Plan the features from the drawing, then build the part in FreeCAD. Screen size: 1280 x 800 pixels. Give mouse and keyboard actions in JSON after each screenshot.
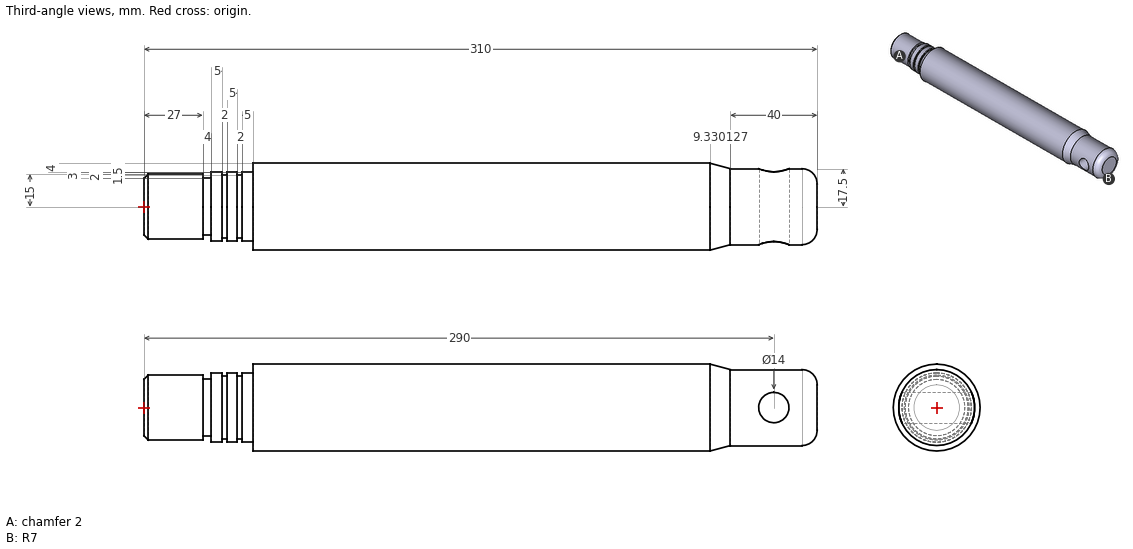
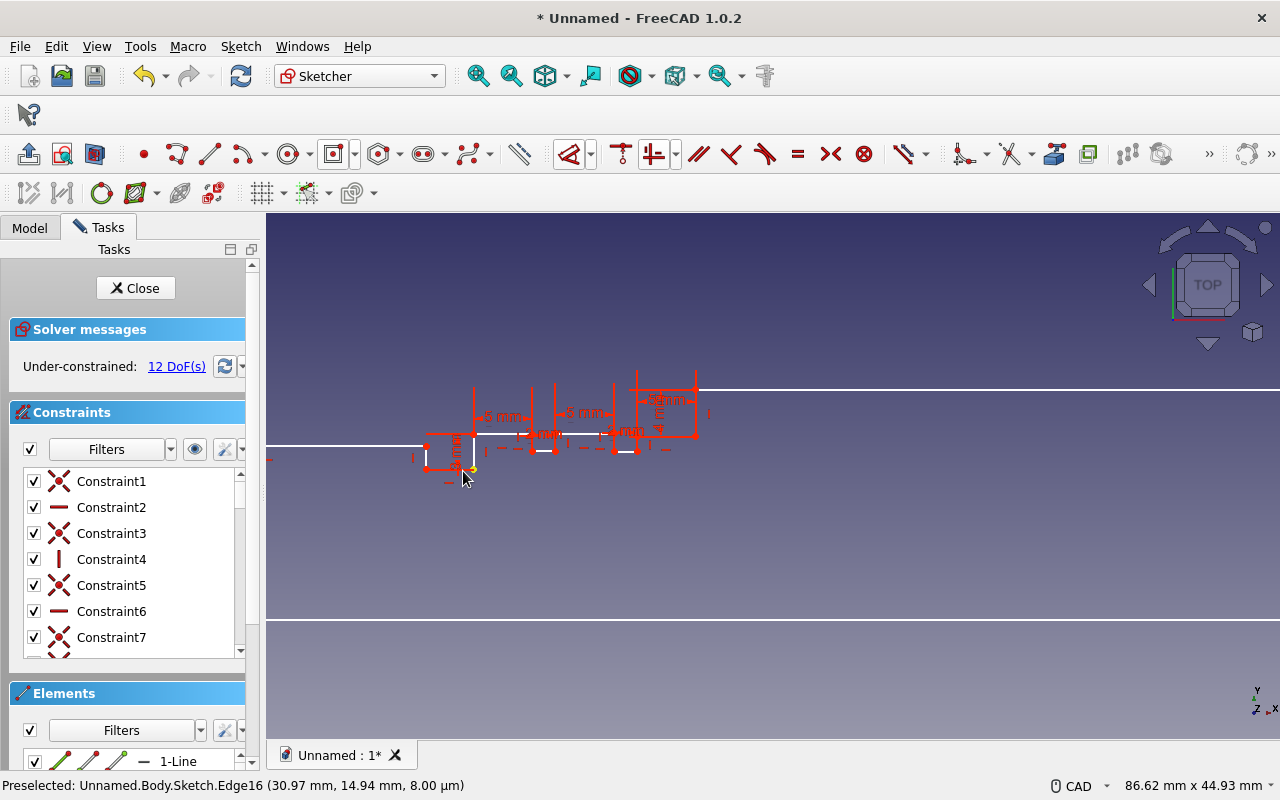
{"action": "left_click", "coordinate": [459, 470]}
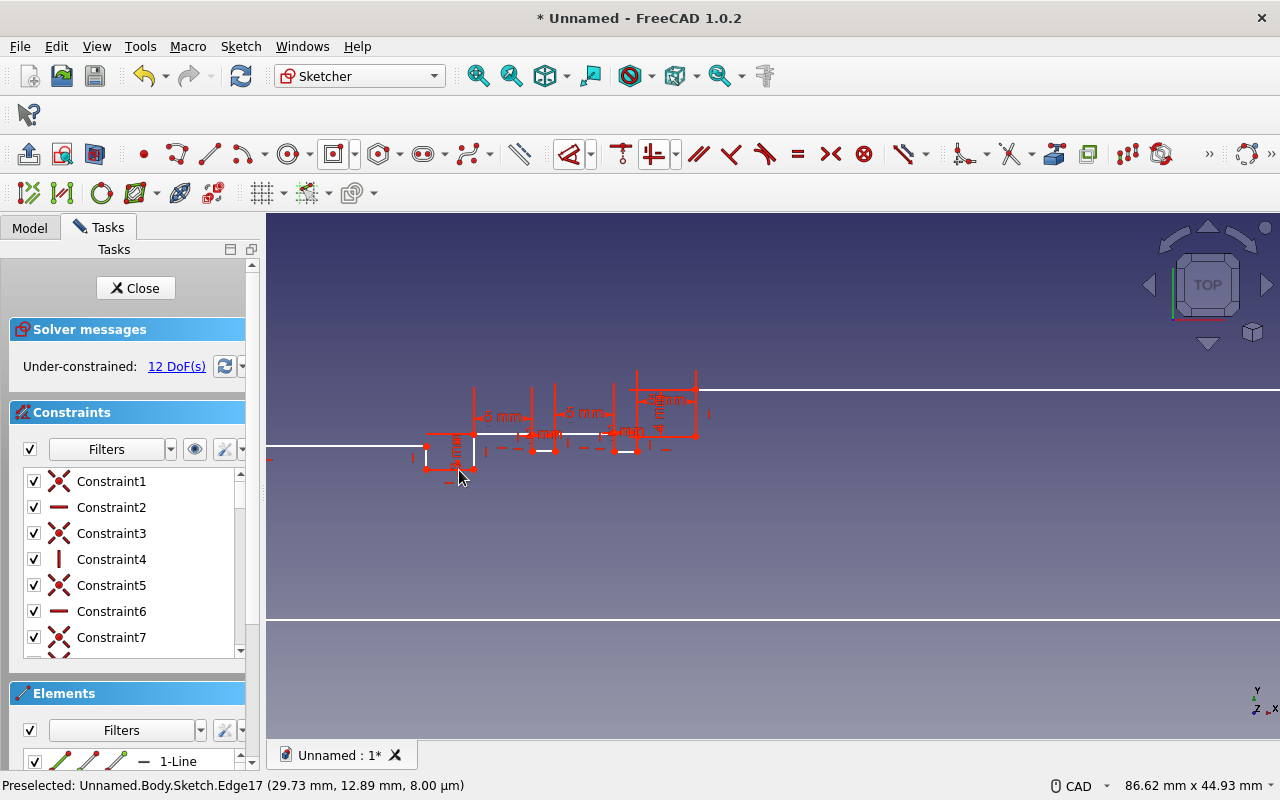
{"action": "key", "text": "l"}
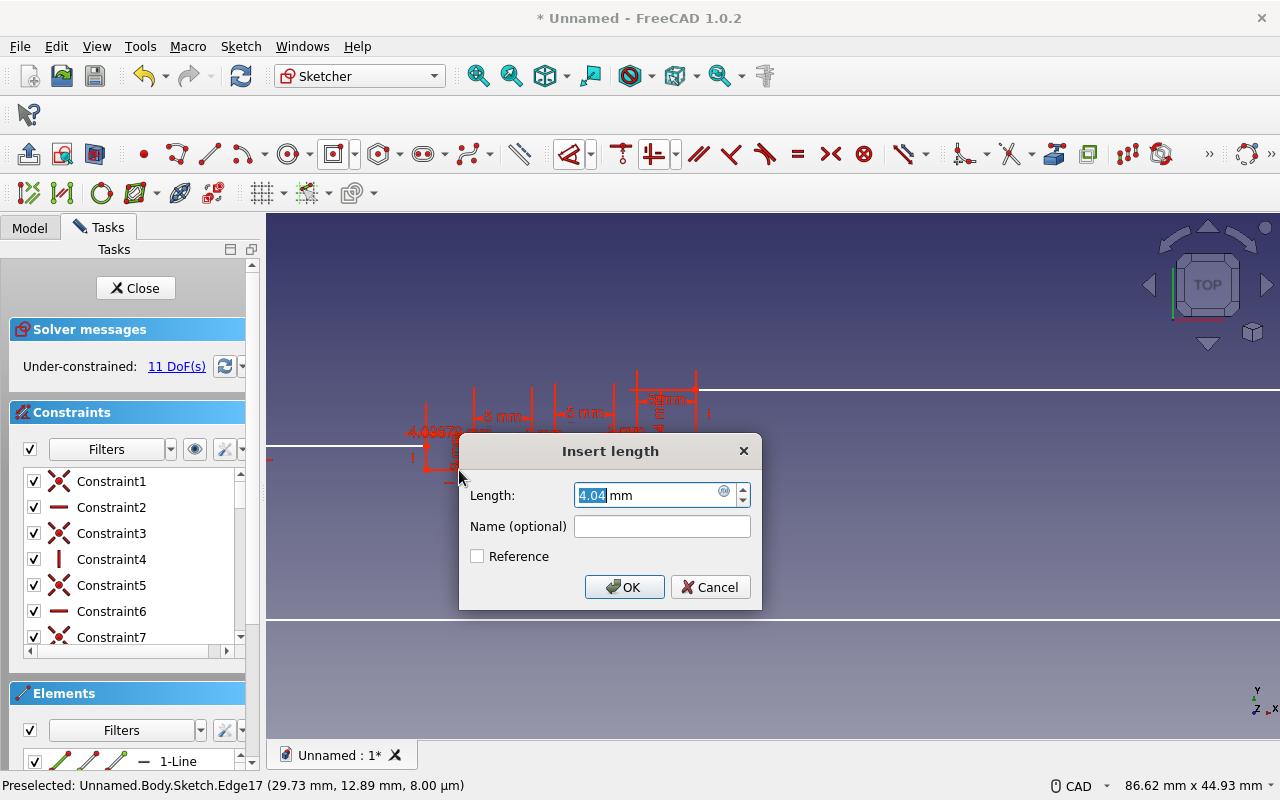
{"action": "type", "text": "4"}
{"action": "key", "text": "Return"}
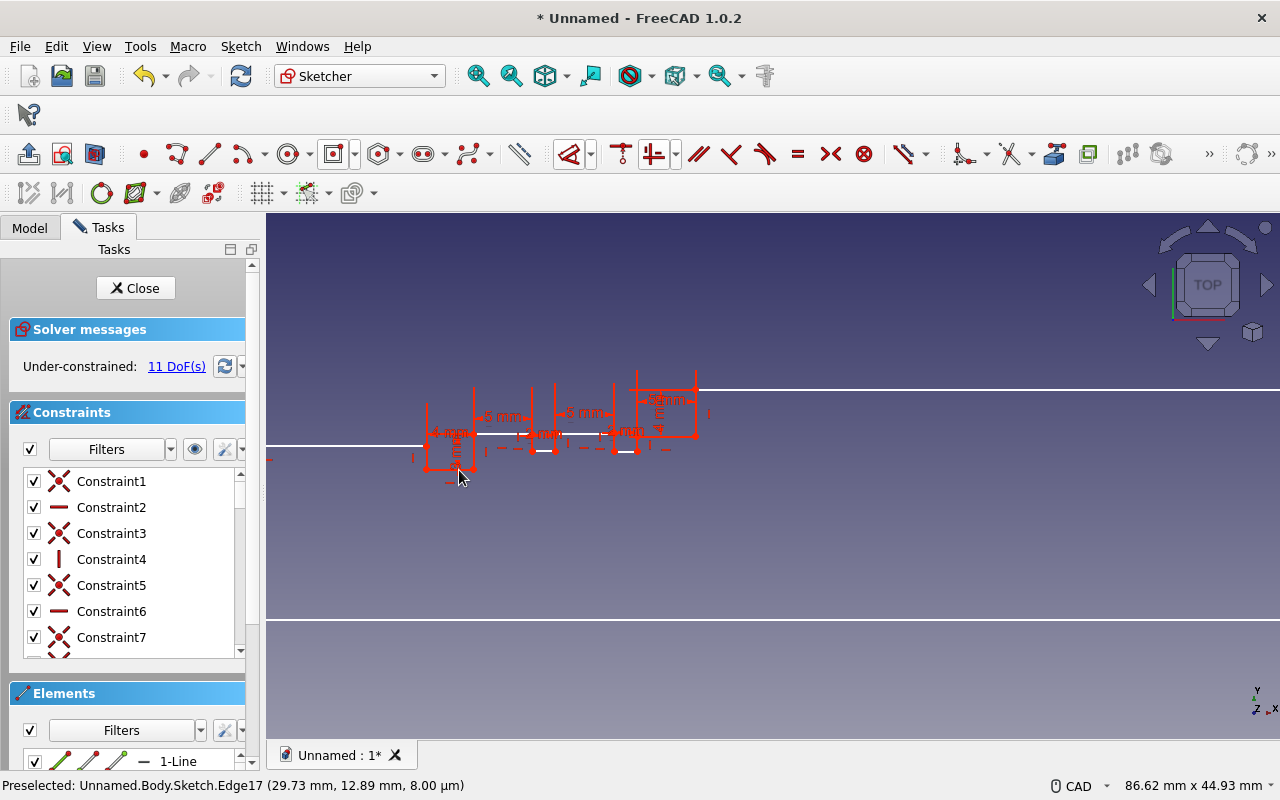
{"action": "scroll", "coordinate": [427, 460], "scroll_direction": "up", "scroll_amount": 3}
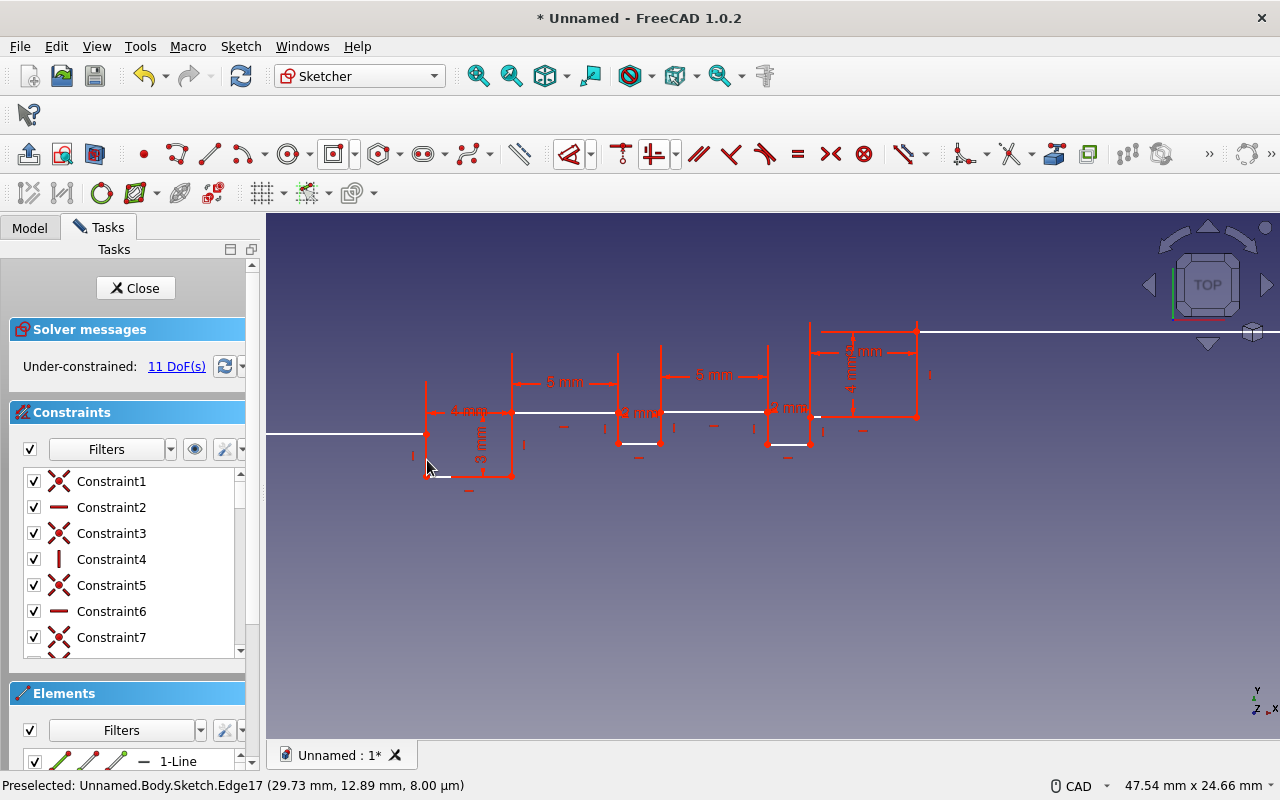
{"action": "left_click", "coordinate": [426, 460]}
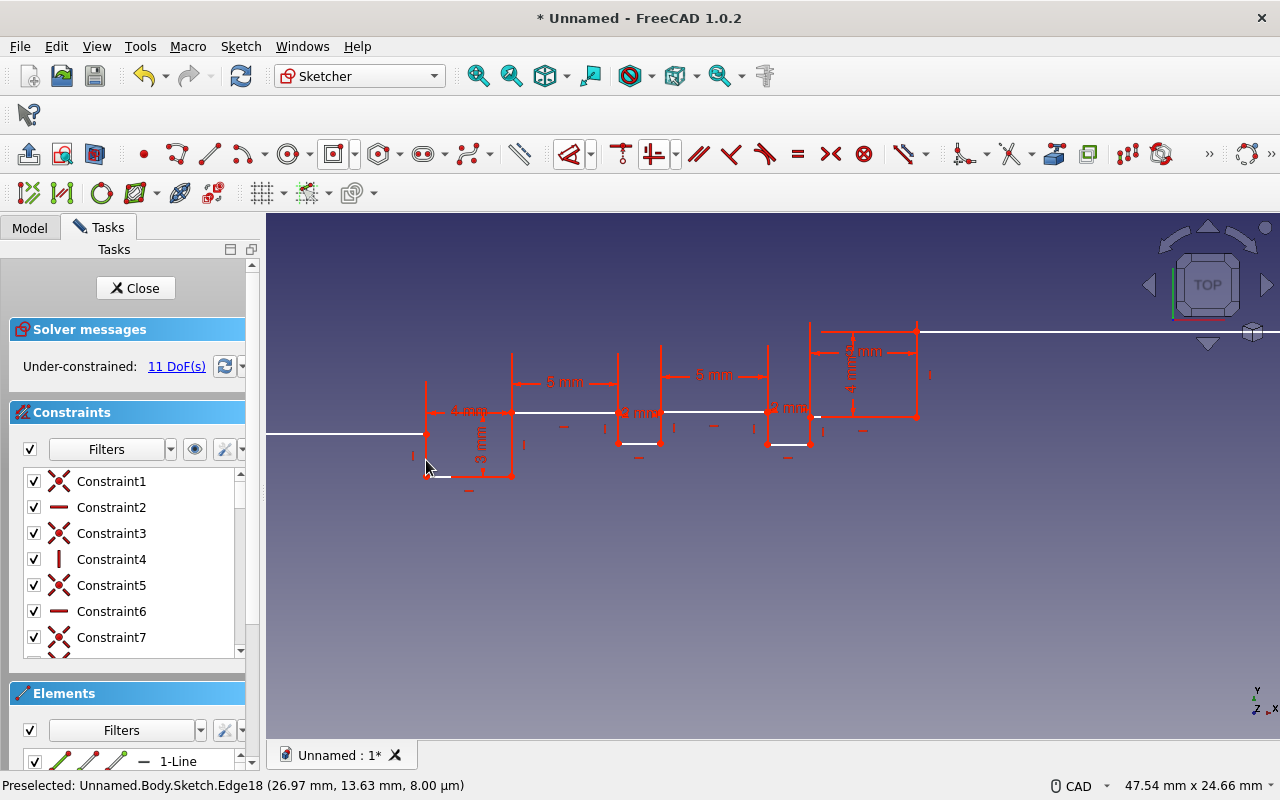
{"action": "key", "text": "i"}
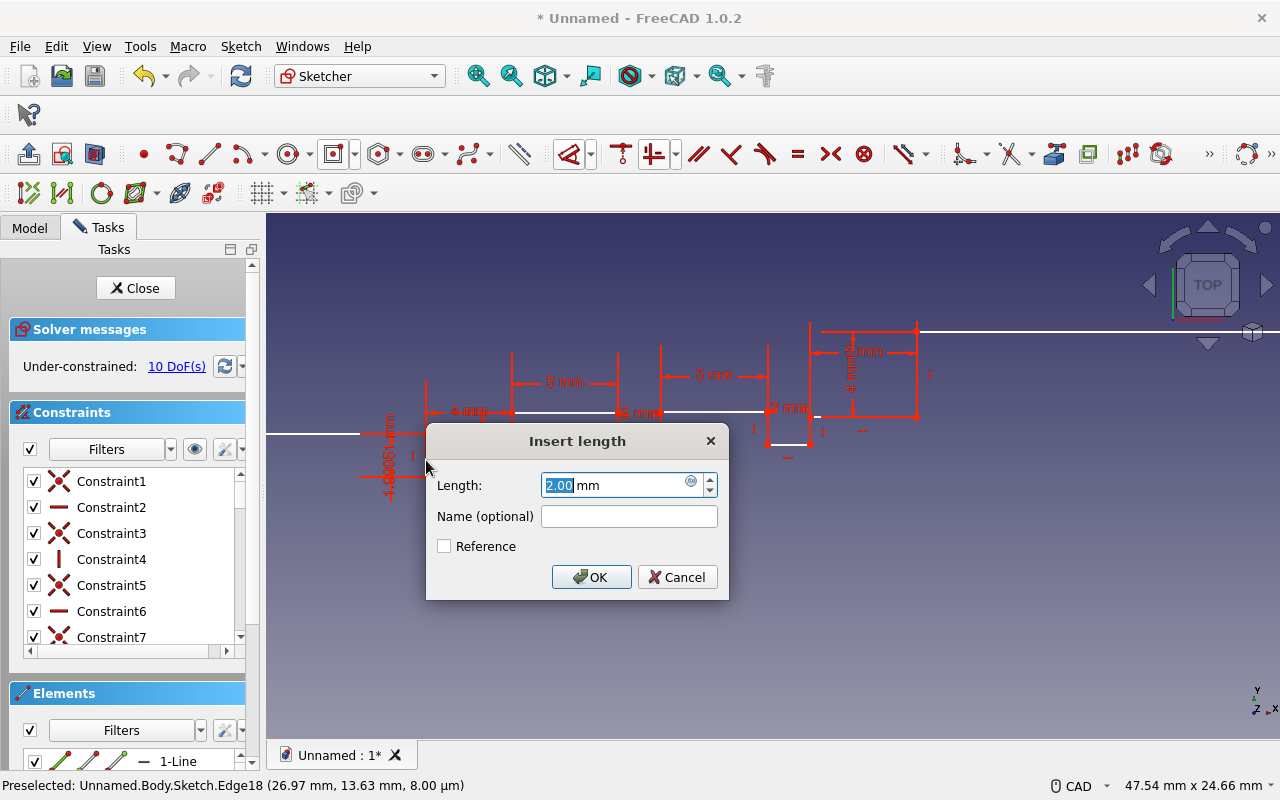
{"action": "type", "text": "2"}
{"action": "key", "text": "Return"}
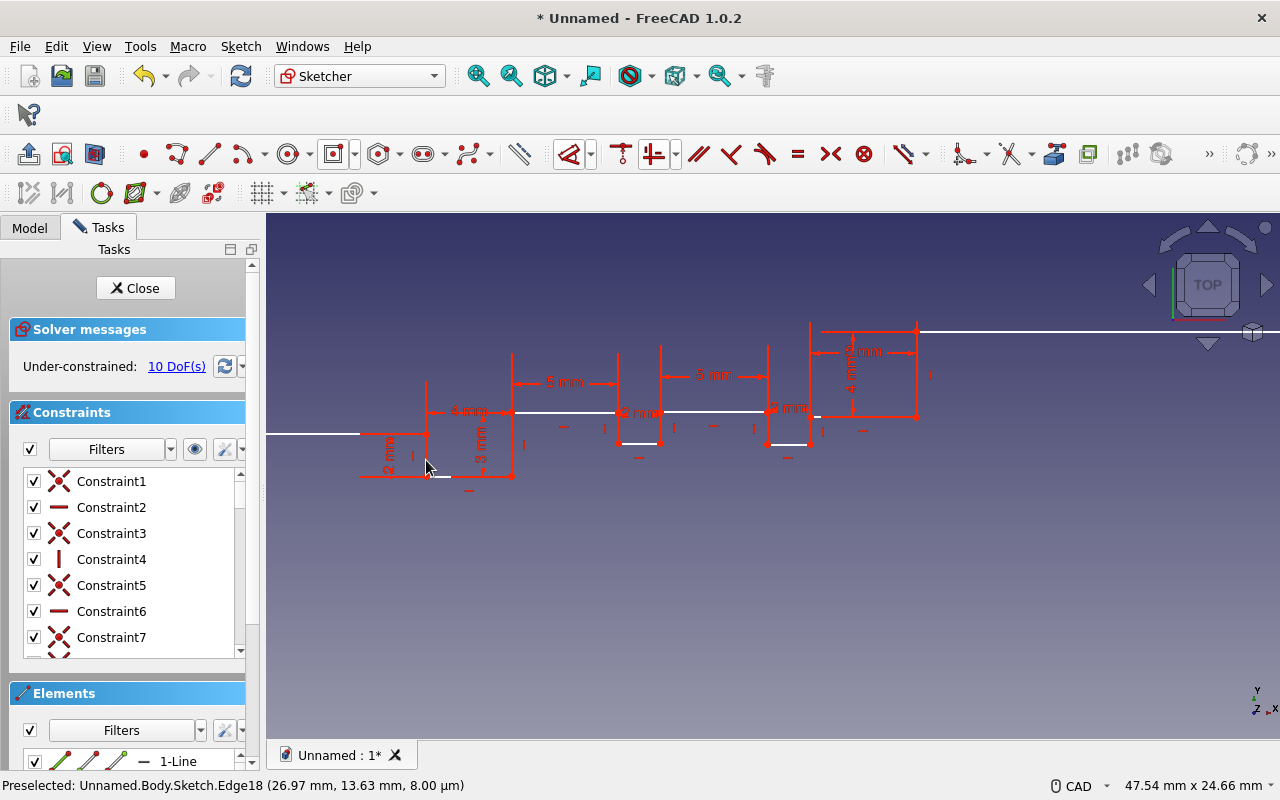
{"action": "scroll", "coordinate": [460, 470], "scroll_direction": "down", "scroll_amount": 12}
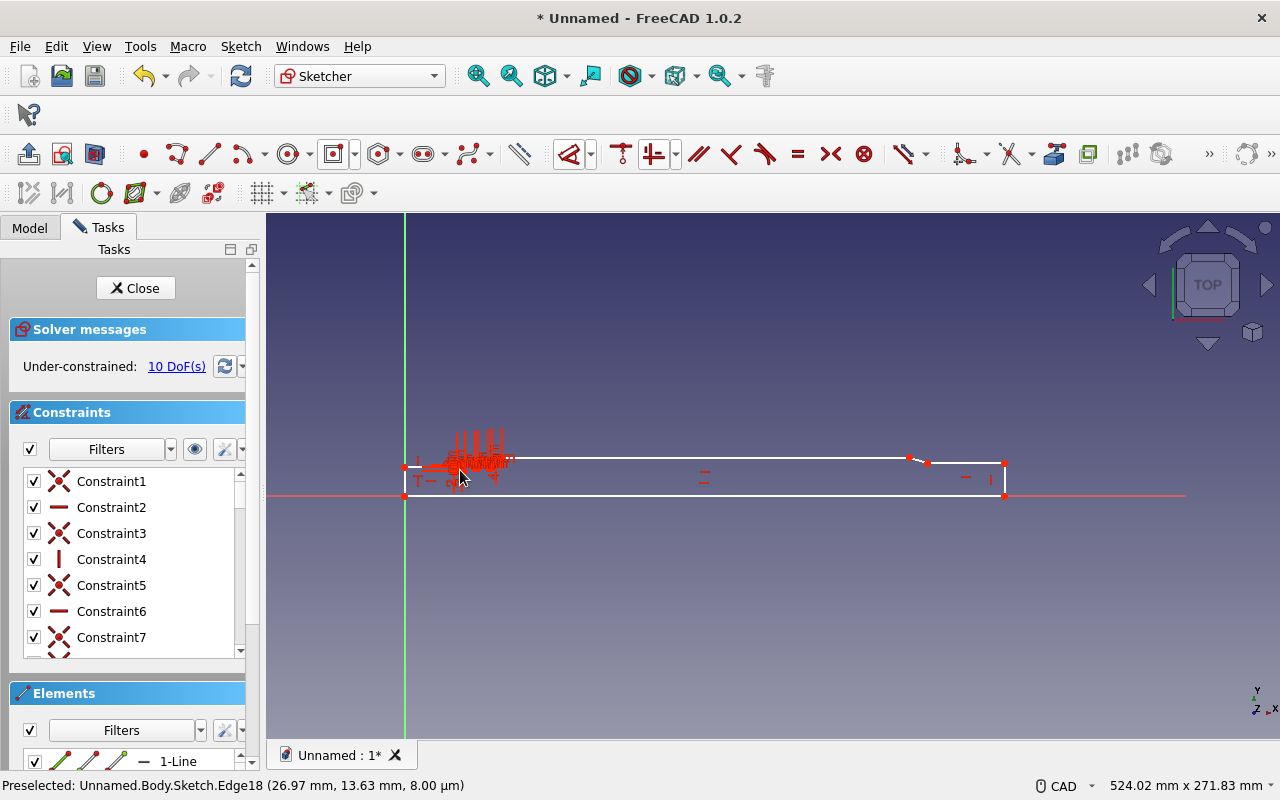
{"action": "left_click", "coordinate": [982, 463]}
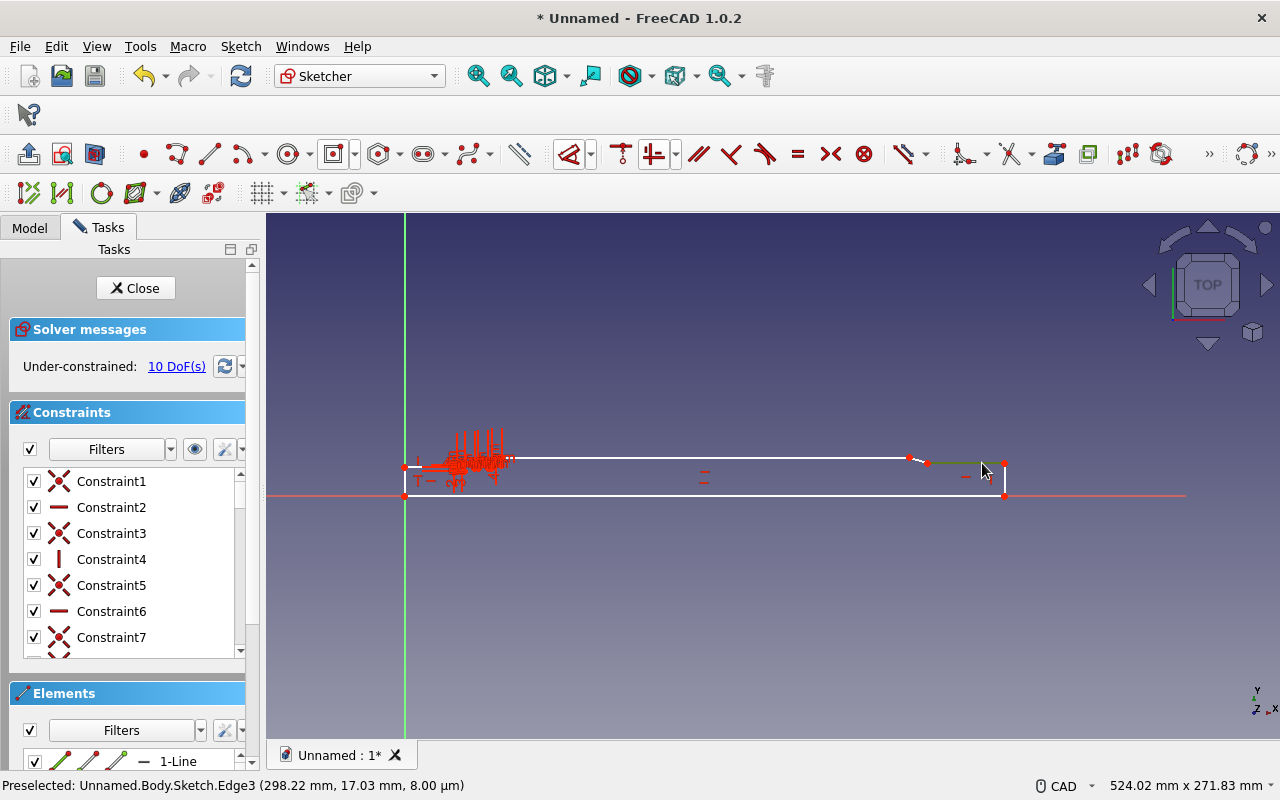
{"action": "left_click", "coordinate": [590, 154]}